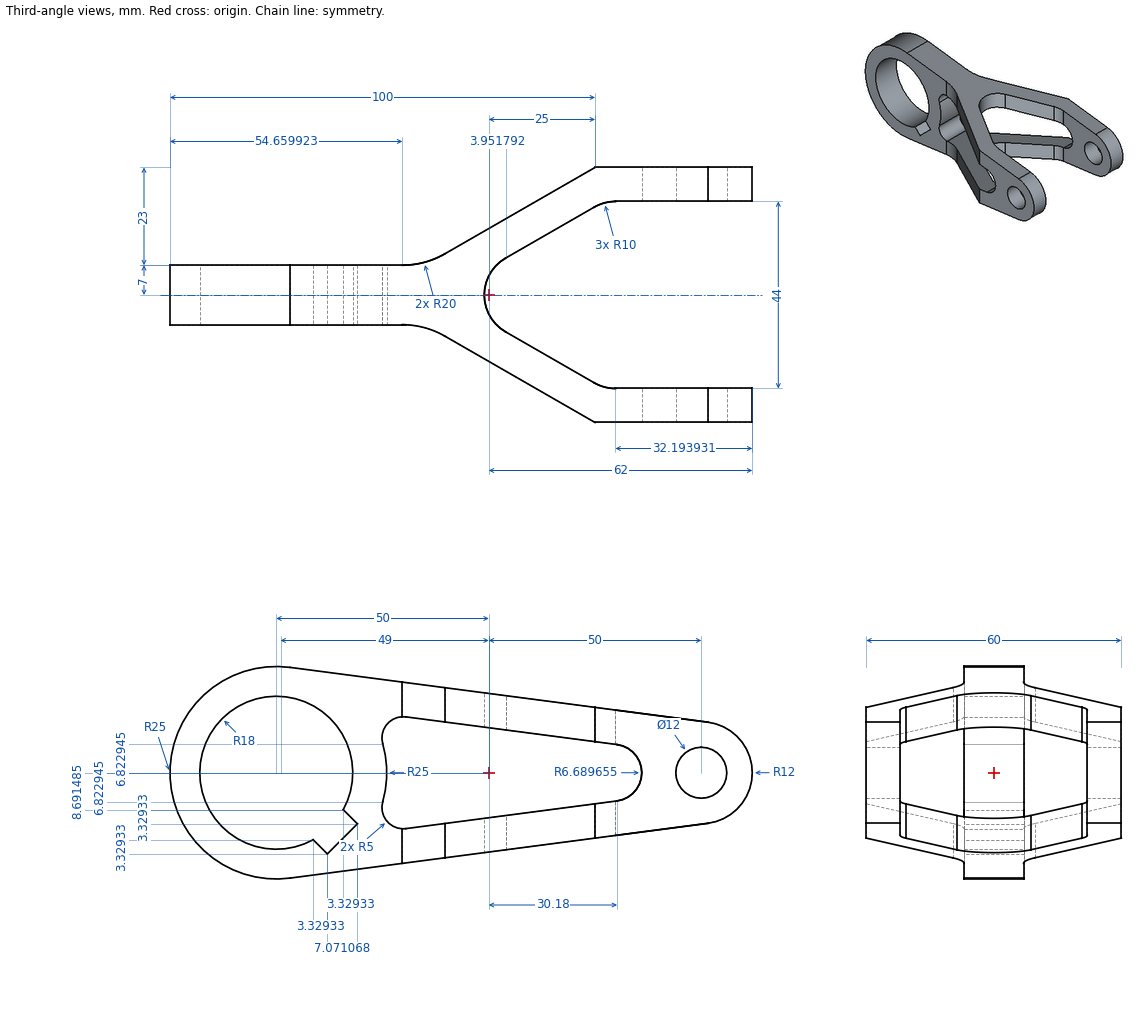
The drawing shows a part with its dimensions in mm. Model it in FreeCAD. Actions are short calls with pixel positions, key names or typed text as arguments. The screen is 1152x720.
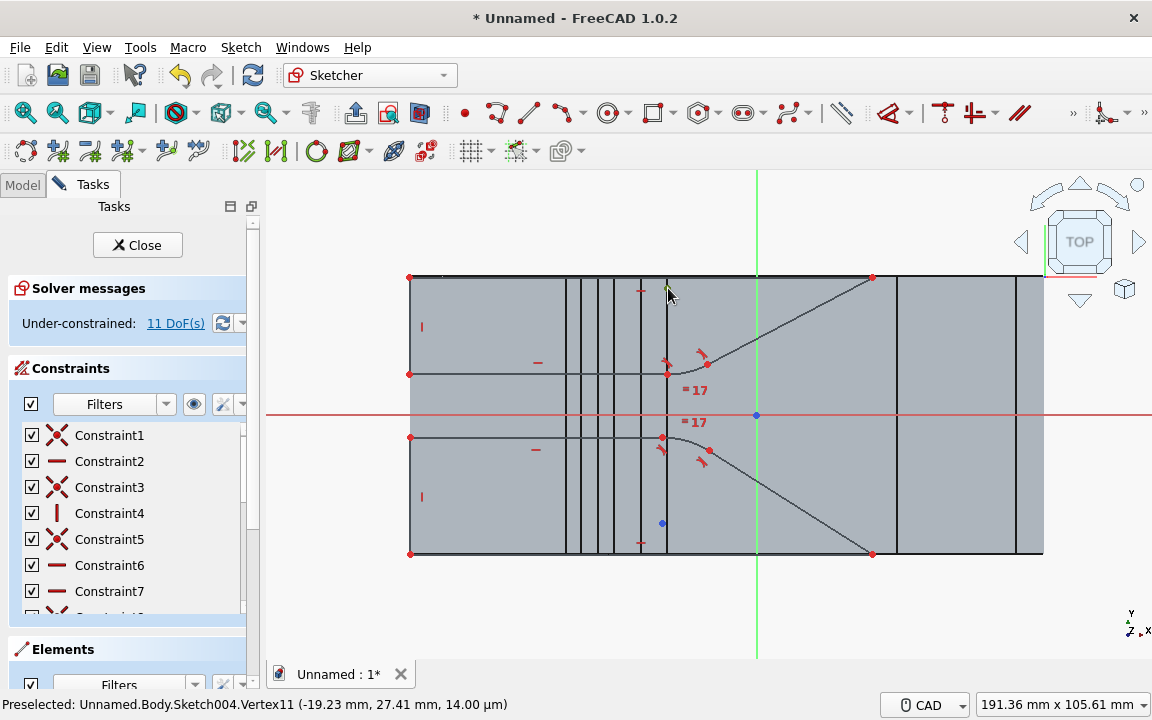
click(663, 524)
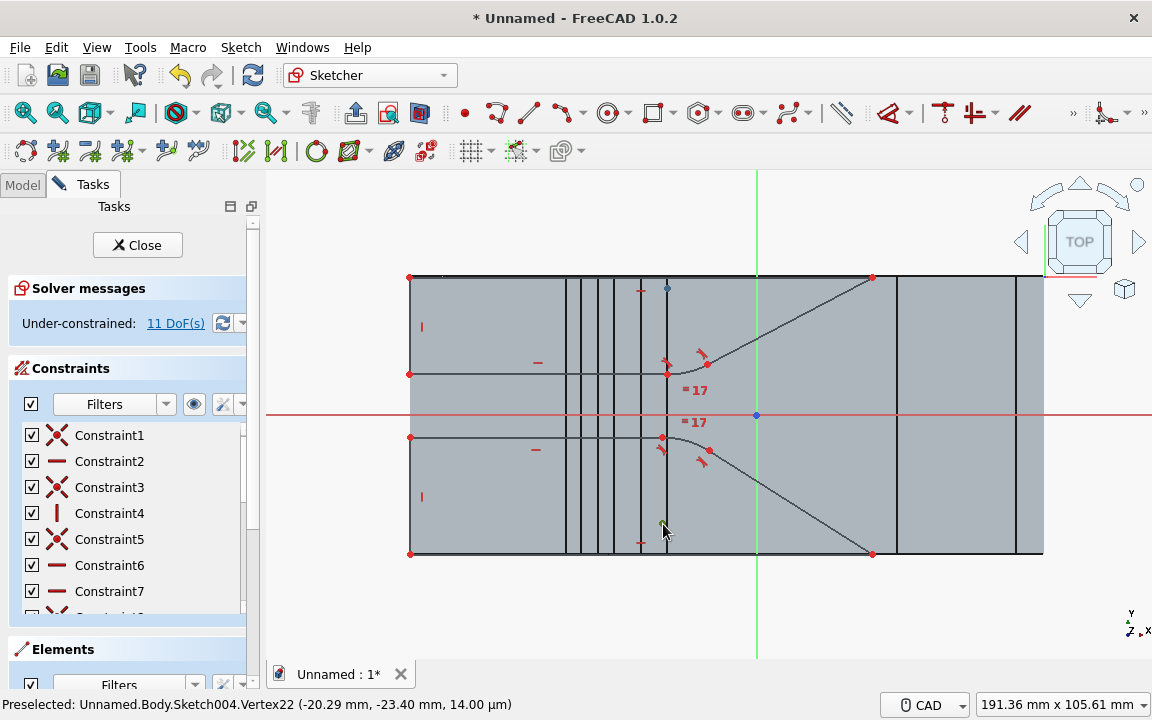
click(344, 415)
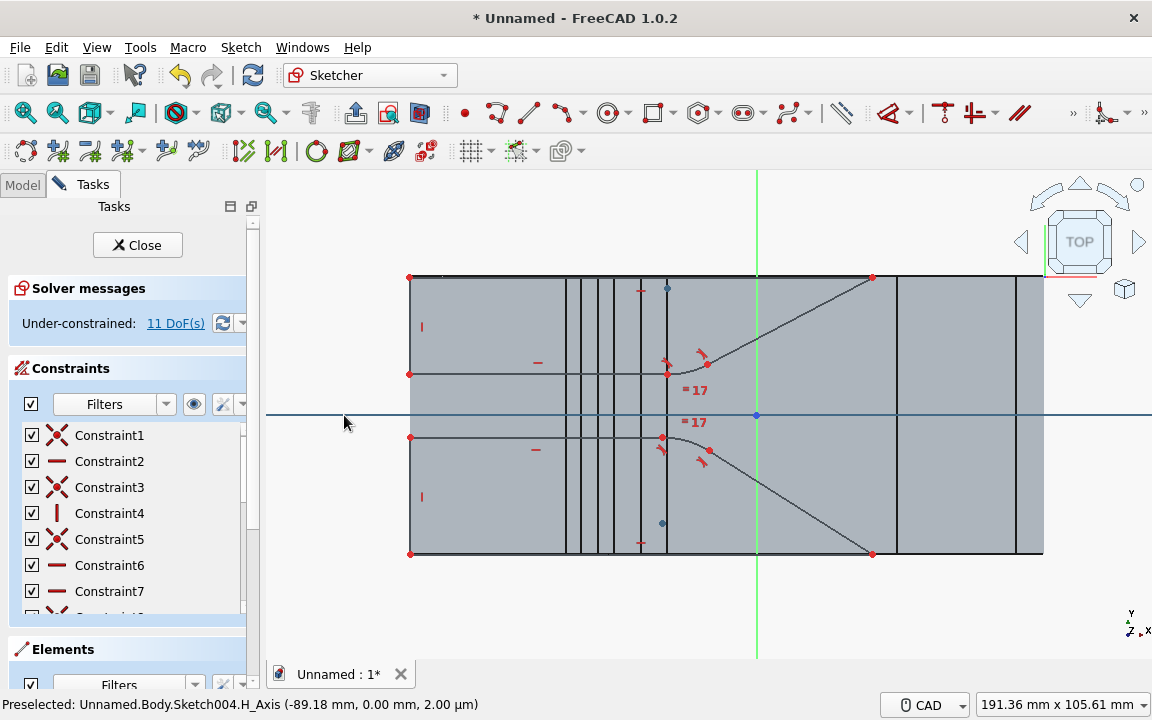
key(s)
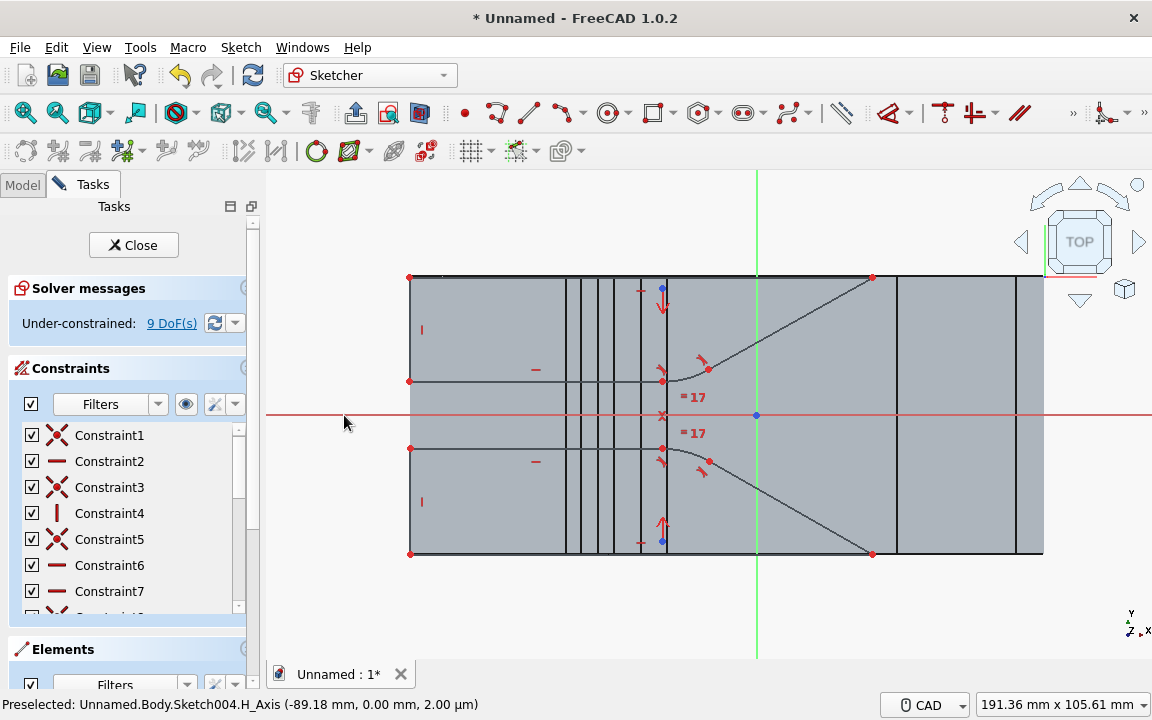
click(410, 278)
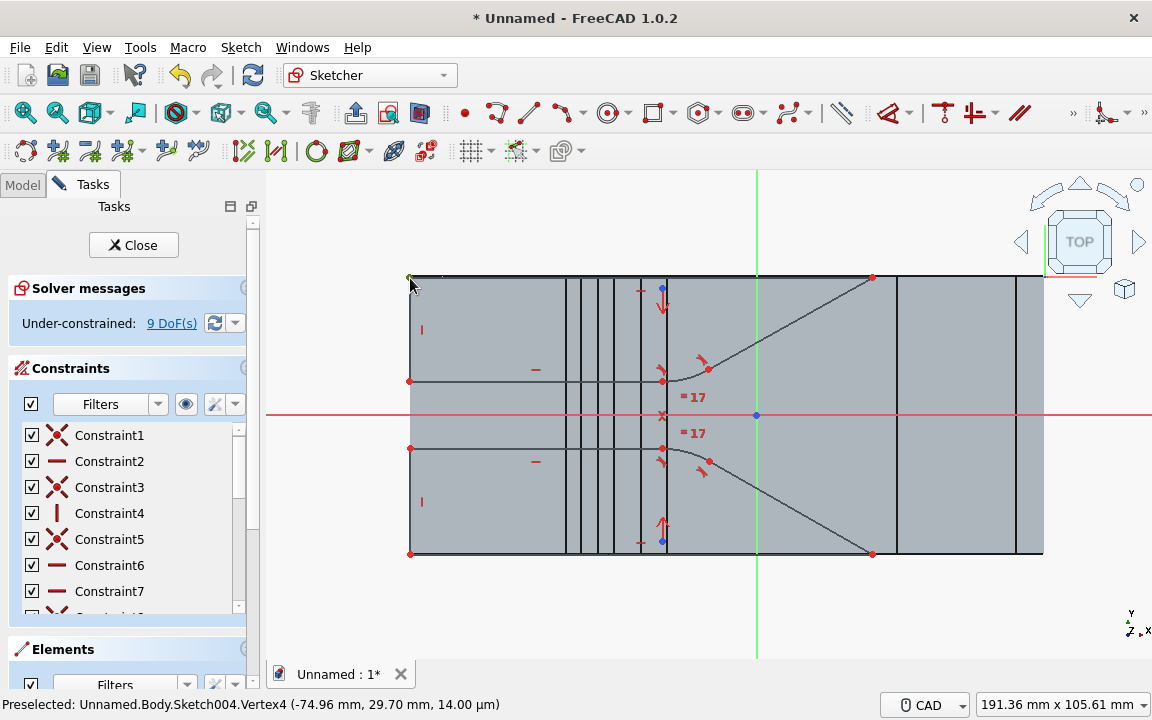
click(410, 555)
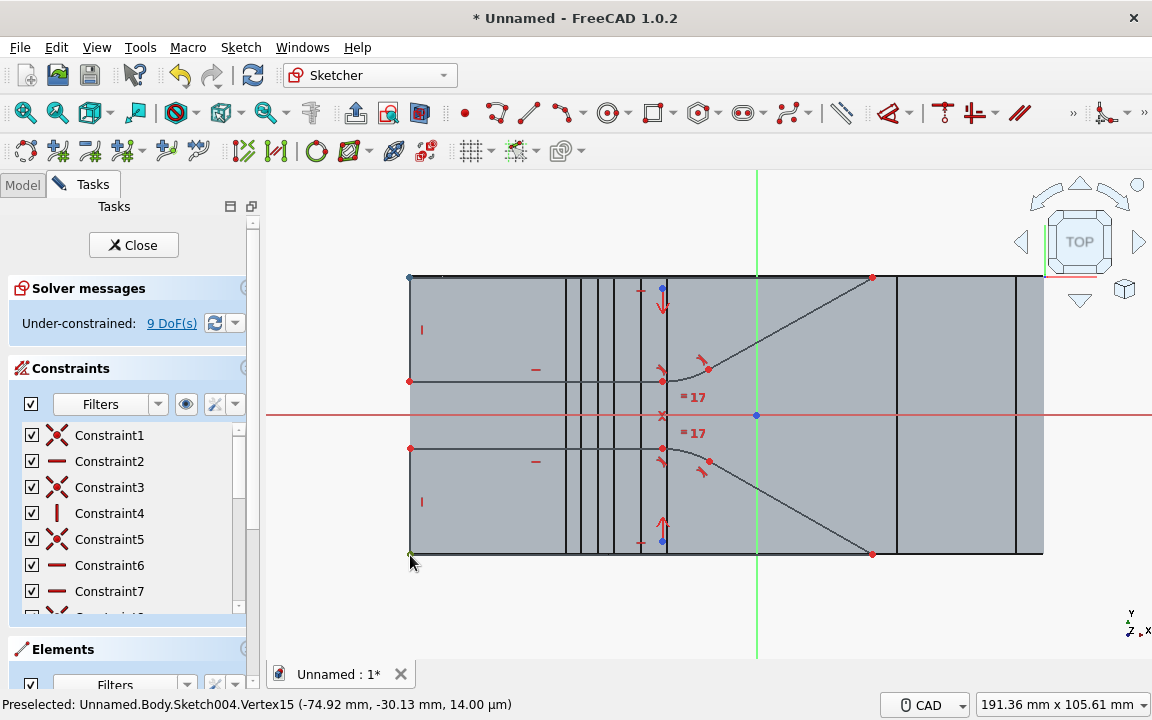
click(344, 415)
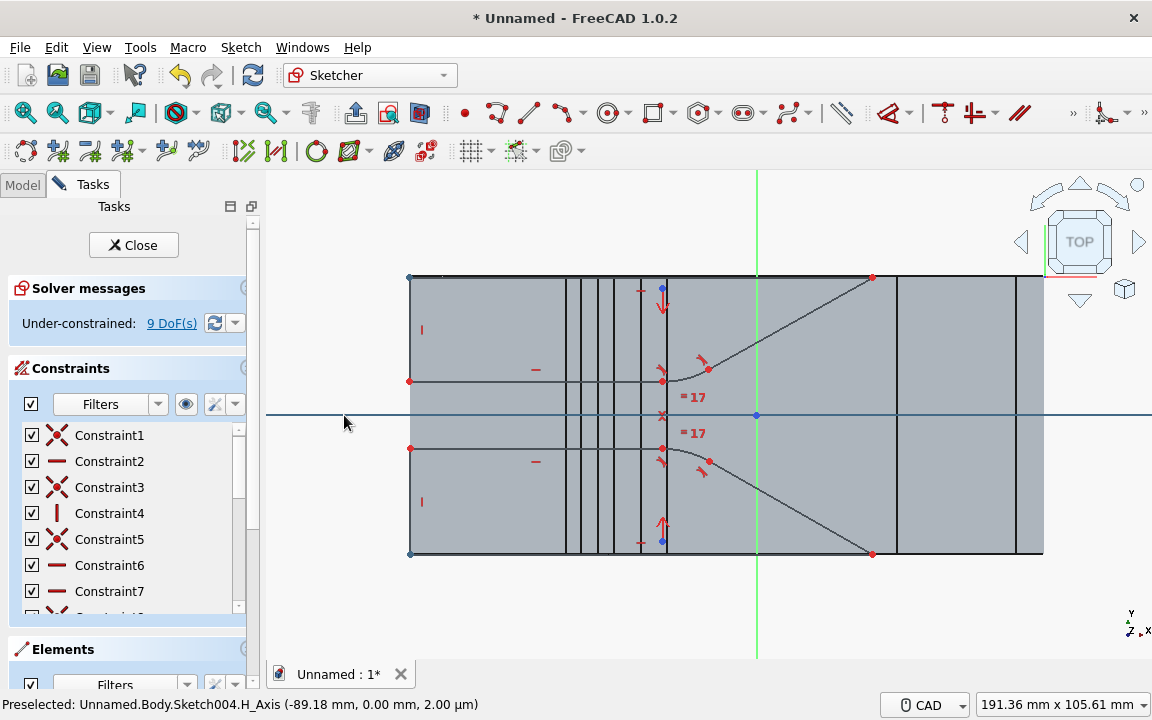
key(s)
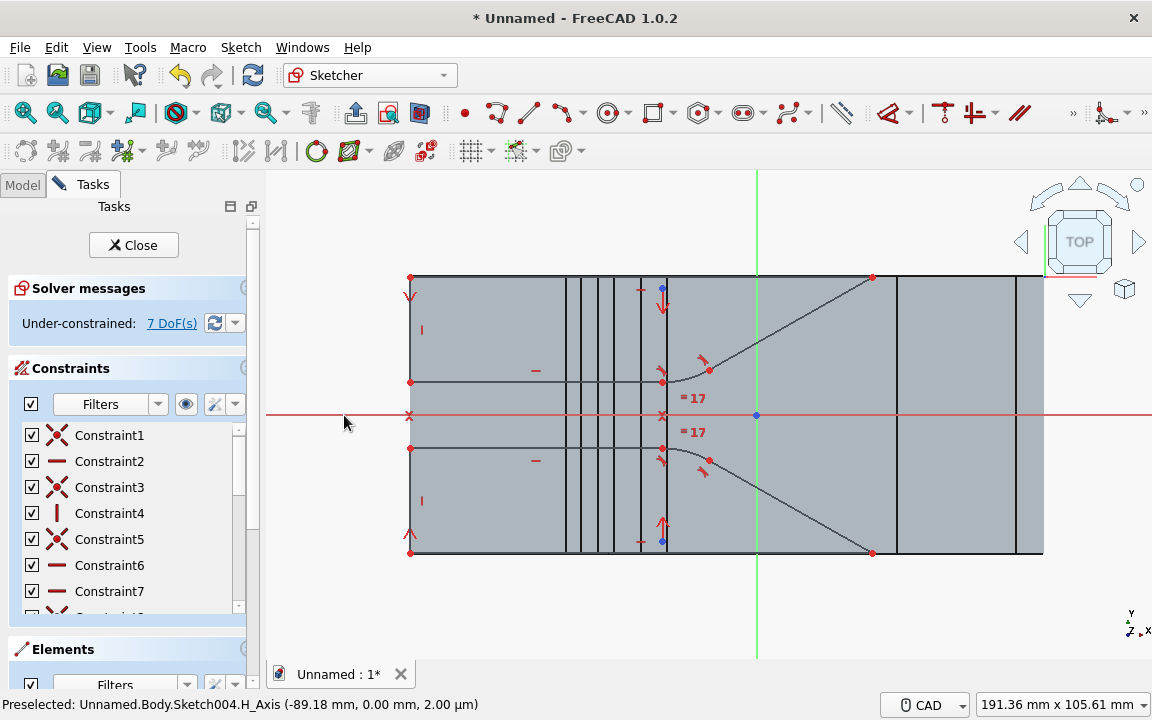
click(888, 114)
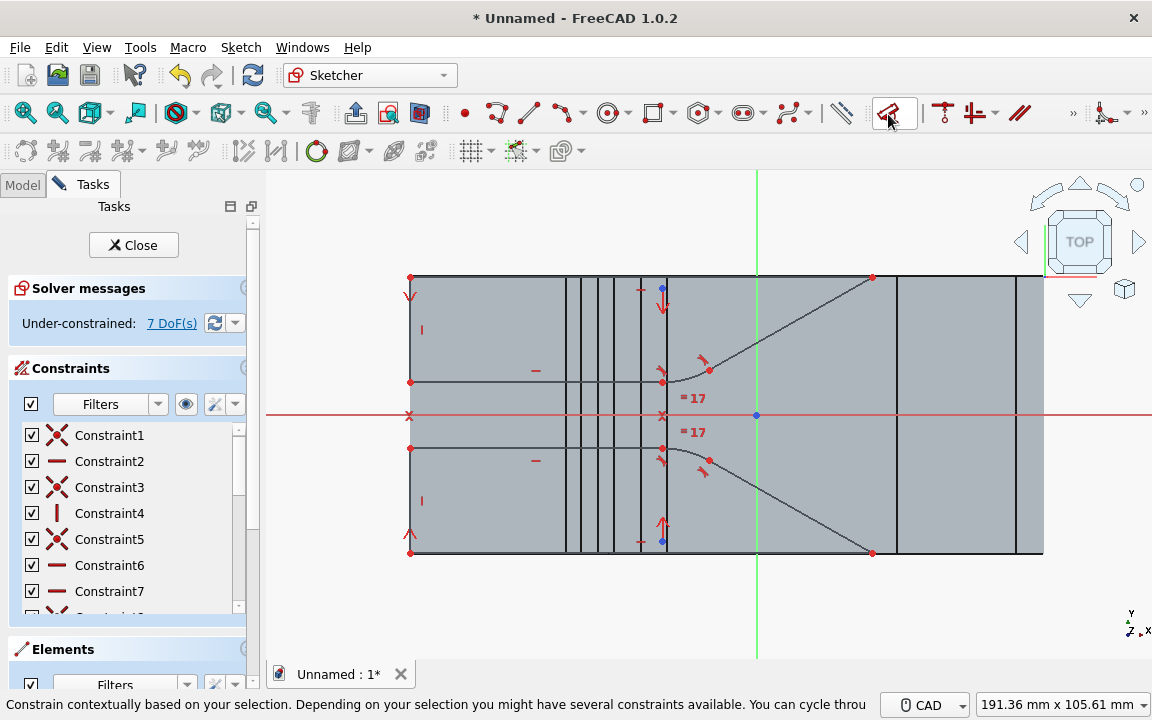
click(677, 381)
click(739, 388)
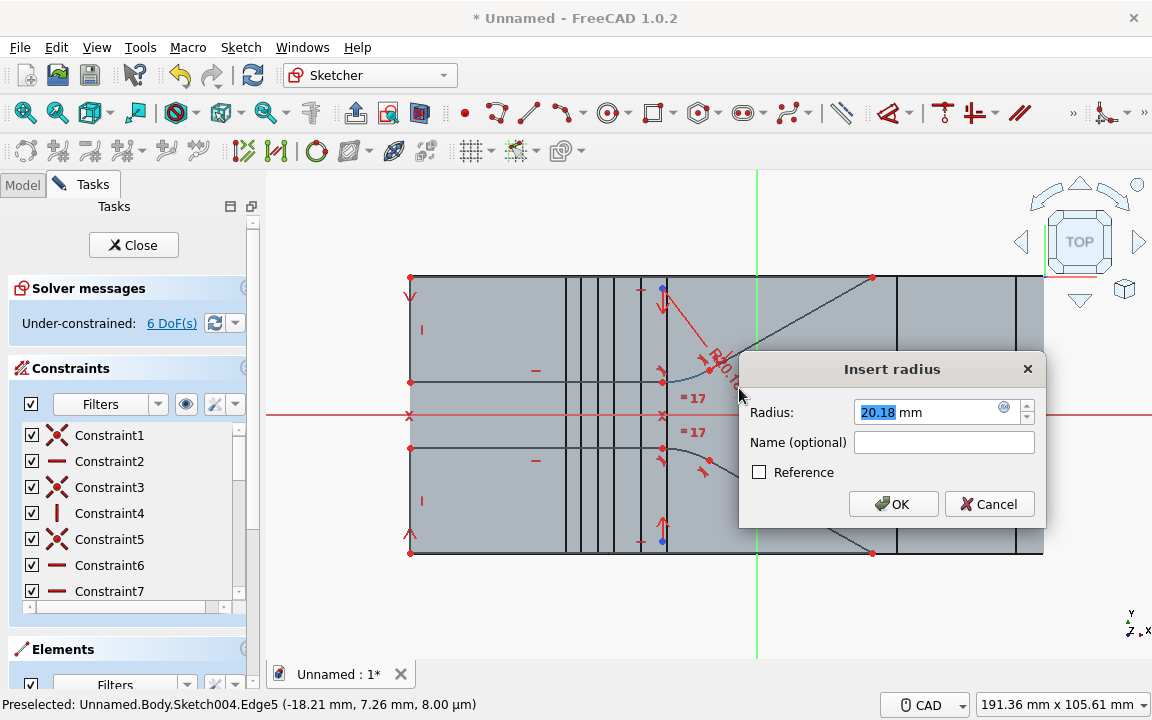
text(20)
key(Return)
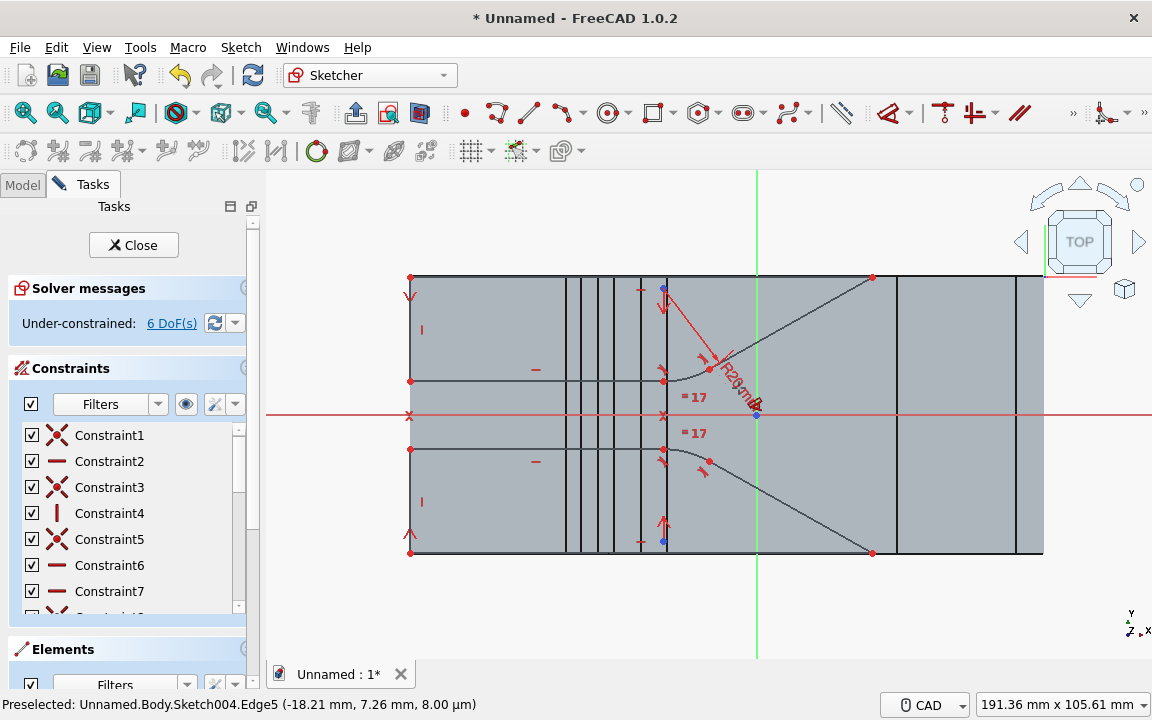
click(410, 308)
click(376, 329)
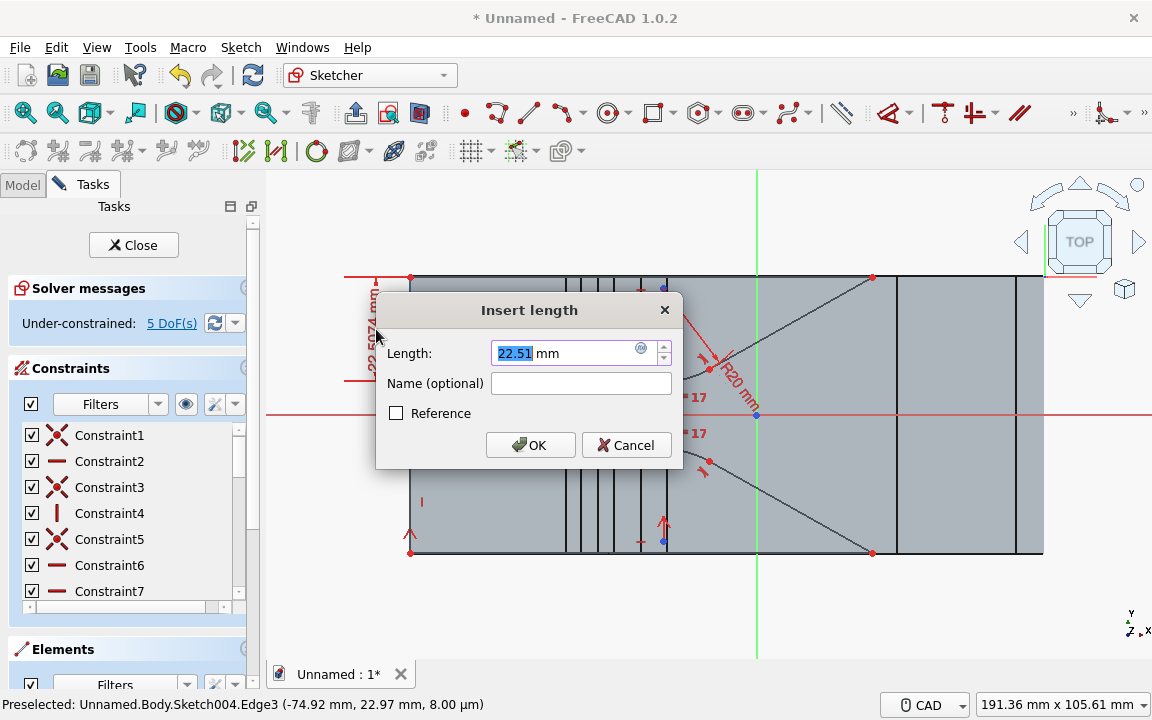
text(23)
key(Return)